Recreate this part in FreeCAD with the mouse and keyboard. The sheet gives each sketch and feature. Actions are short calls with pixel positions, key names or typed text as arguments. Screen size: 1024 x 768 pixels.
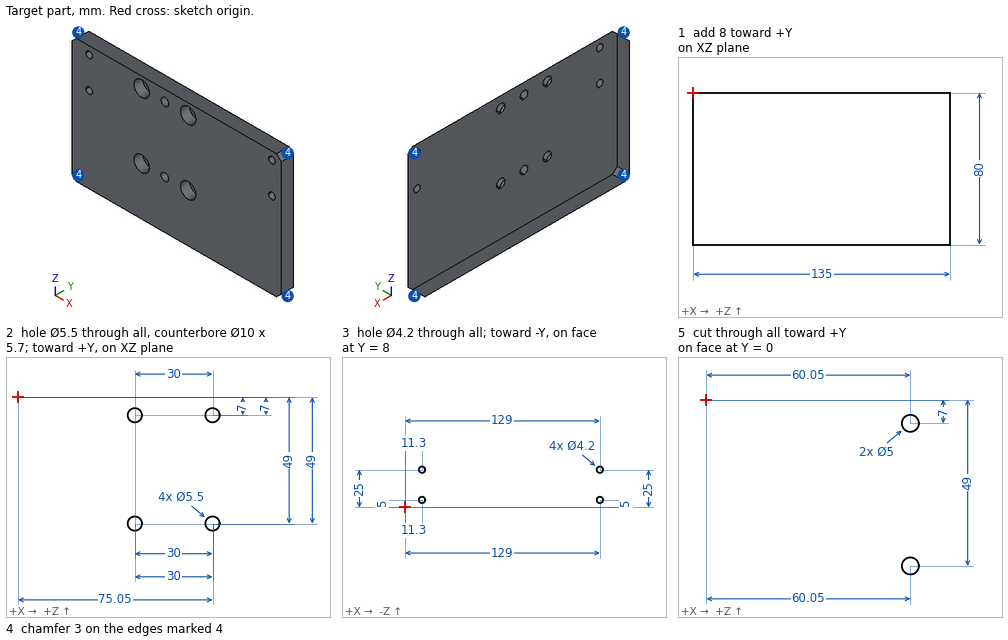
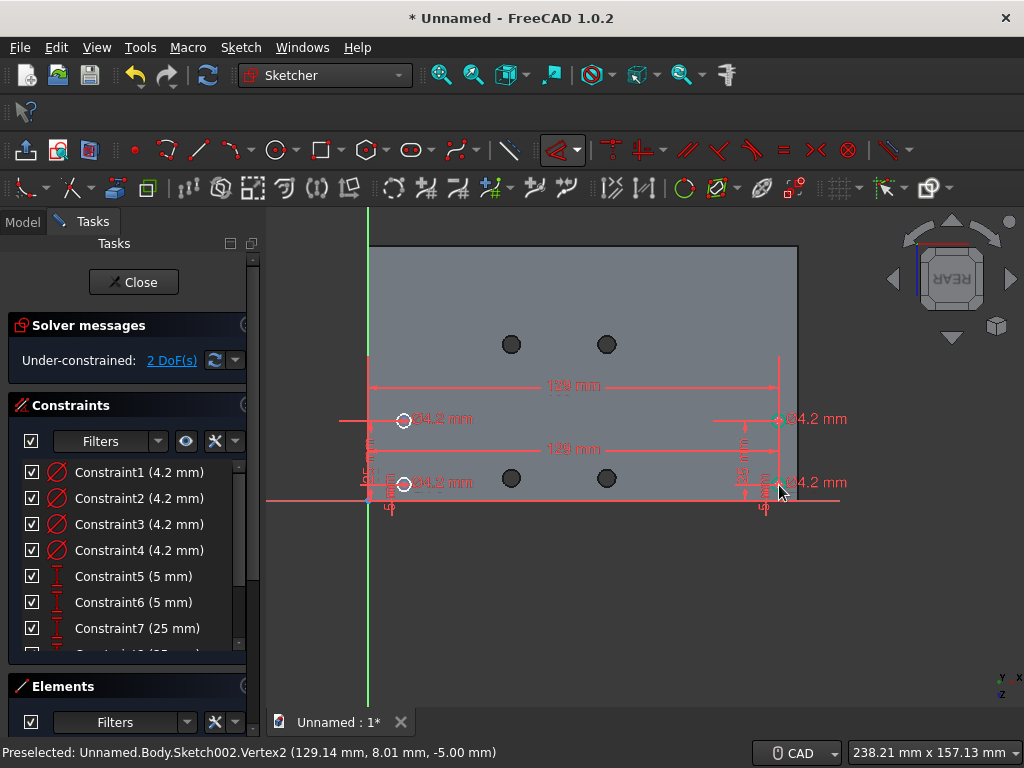
click(404, 421)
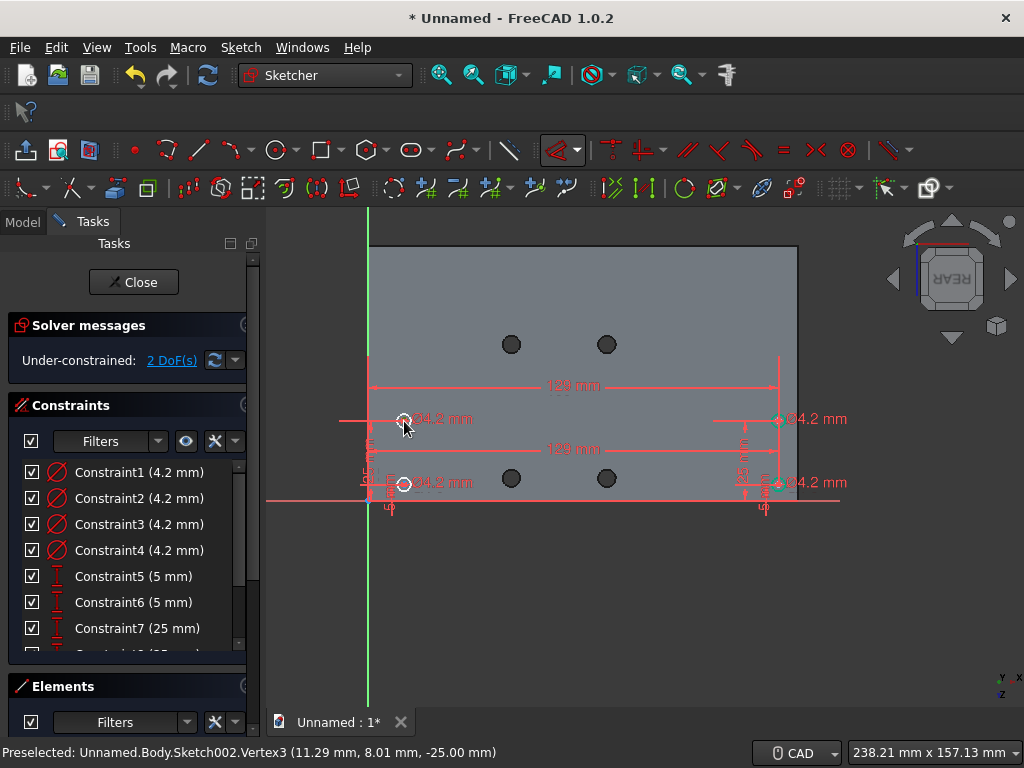
key(l)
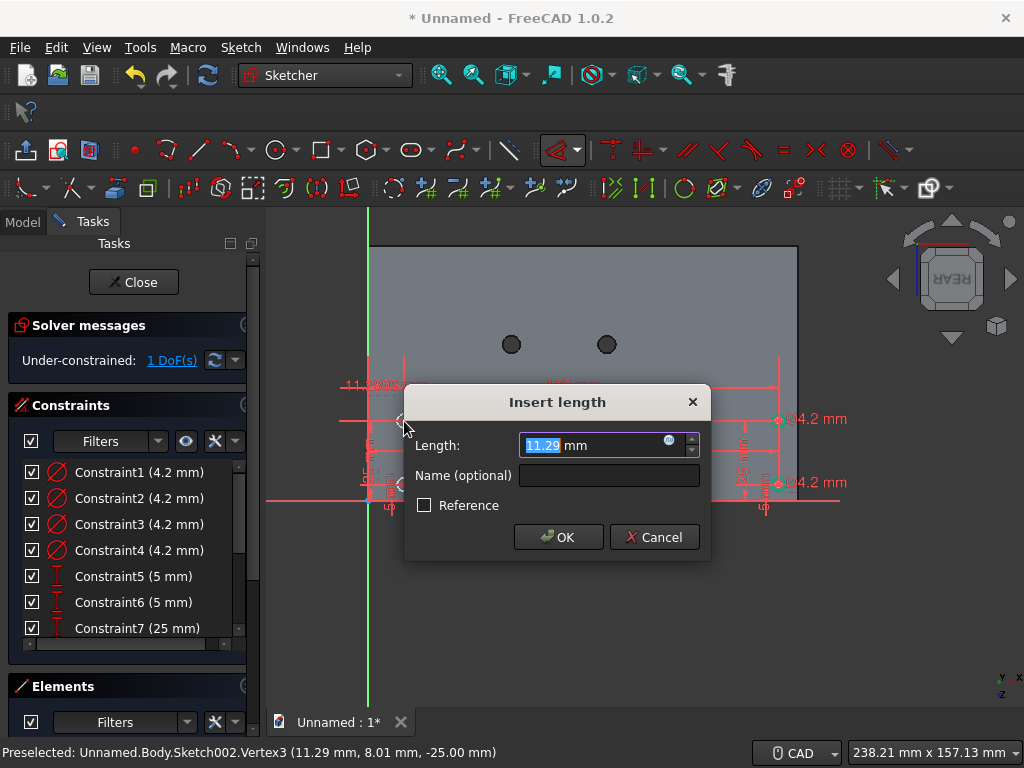
text(11.3)
key(Return)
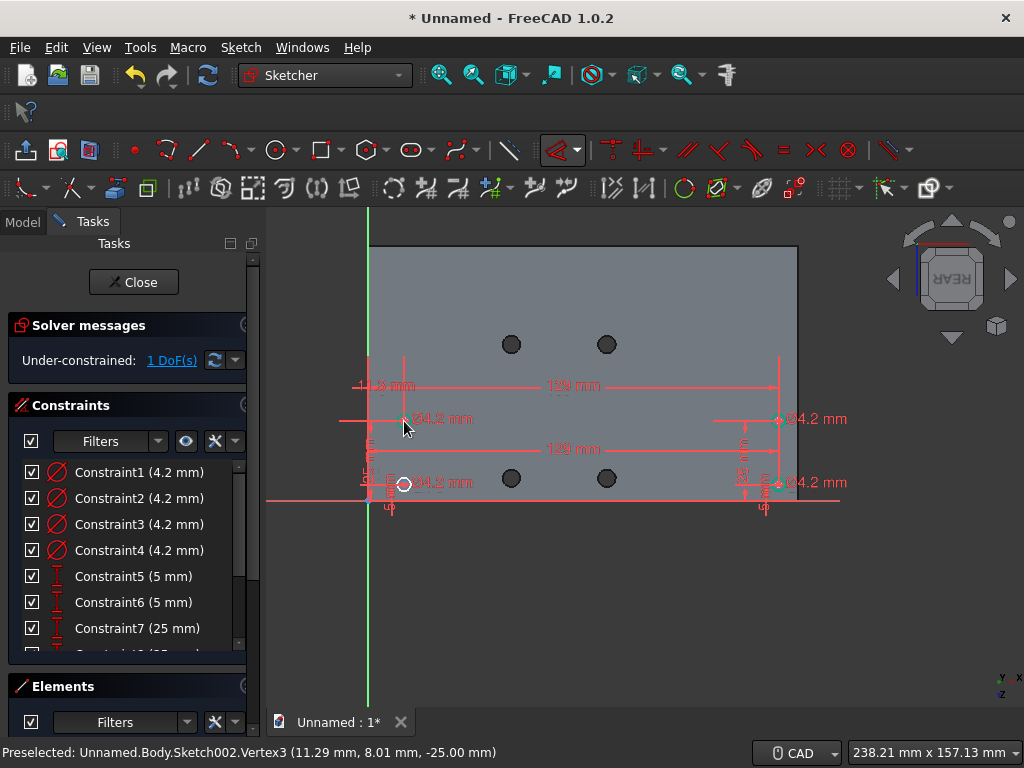
click(404, 485)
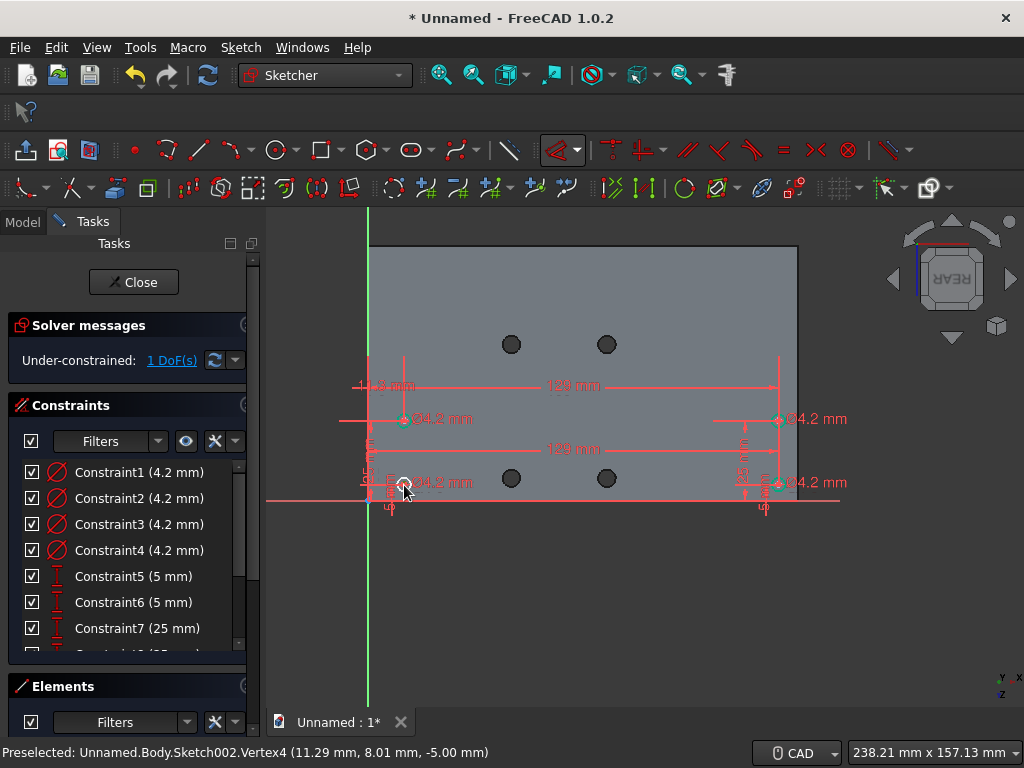
key(l)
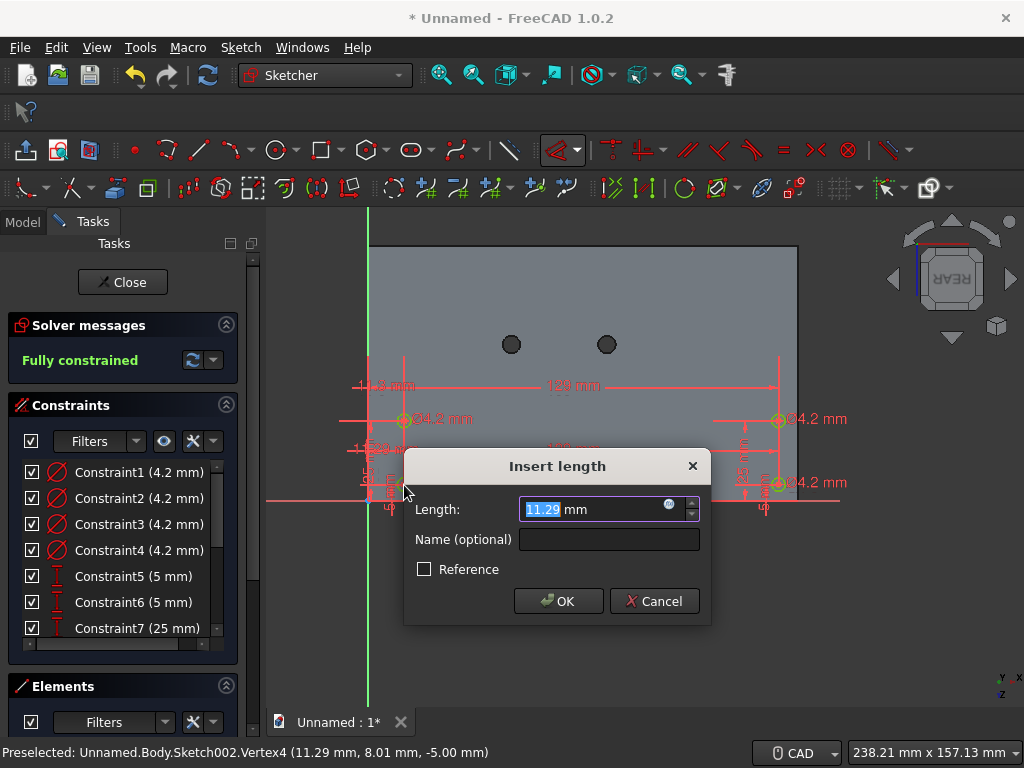
text(11.3)
key(Return)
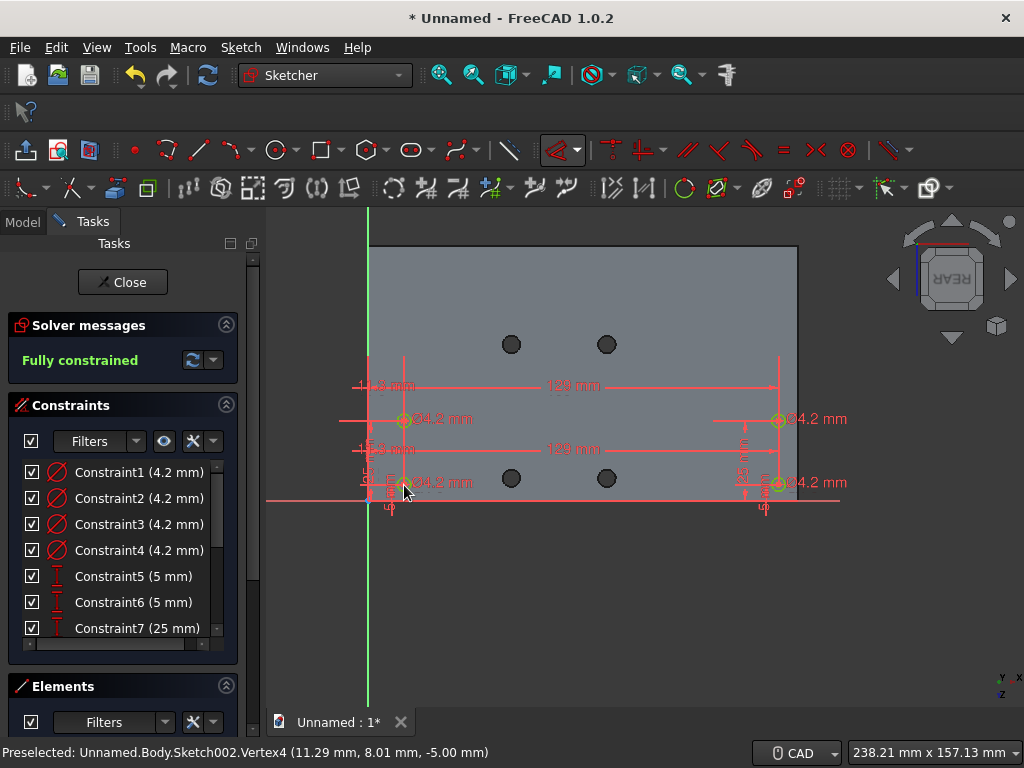
click(123, 282)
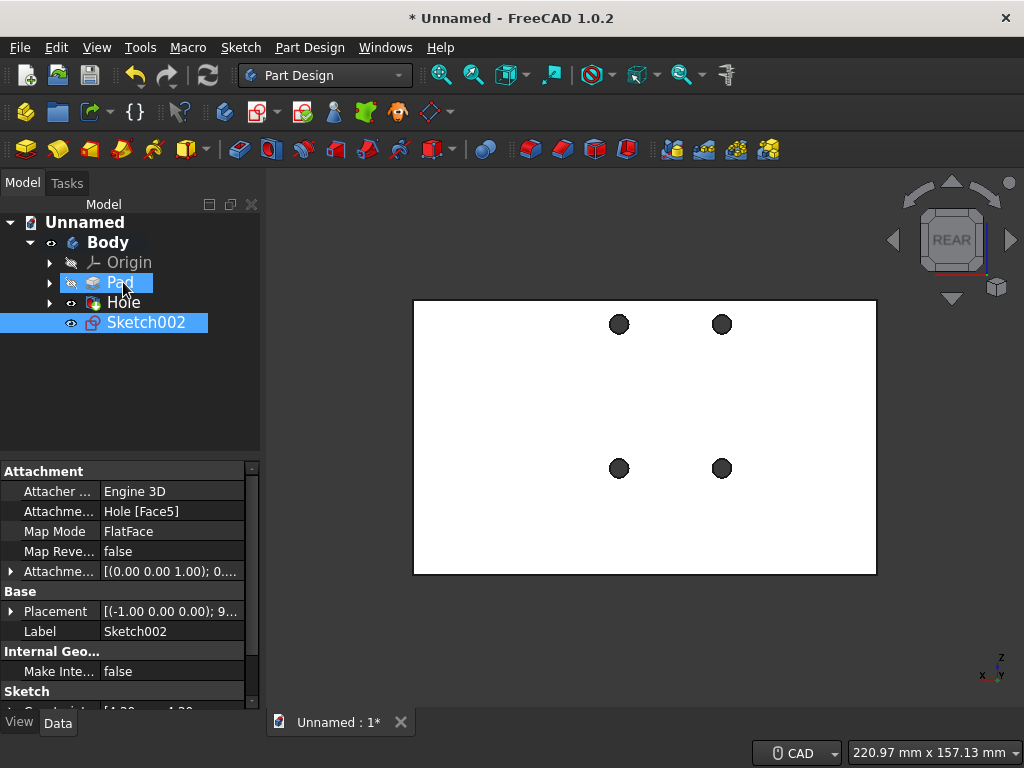
click(272, 150)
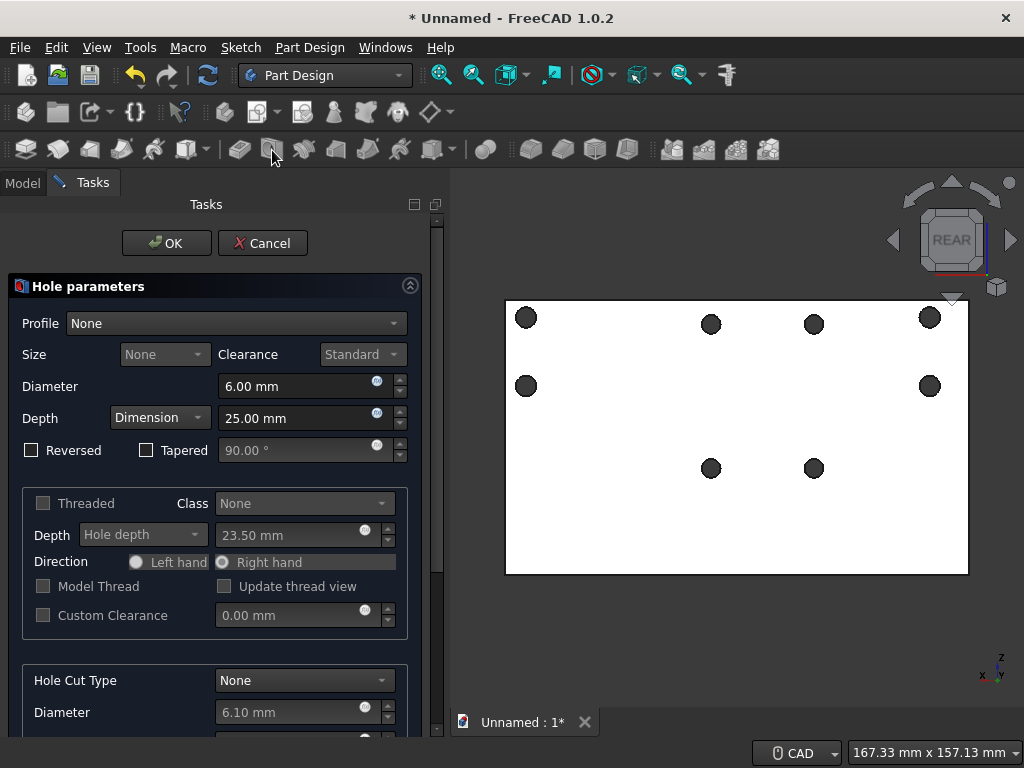
triple_click(305, 386)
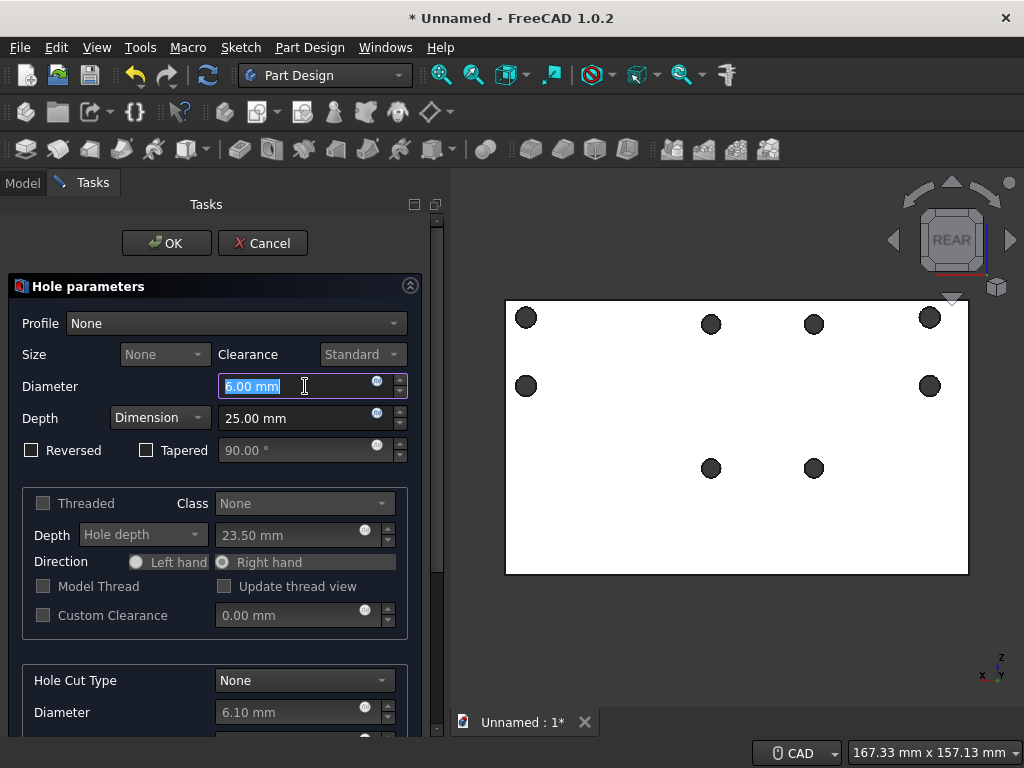
text(4.2)
key(Tab)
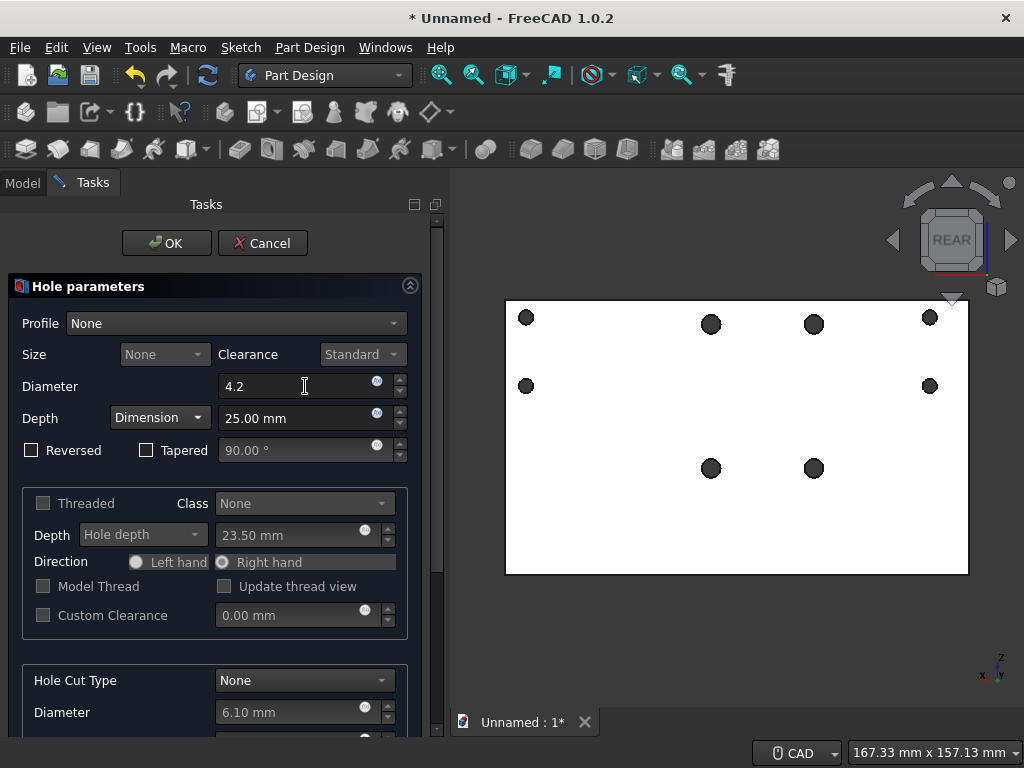
click(161, 418)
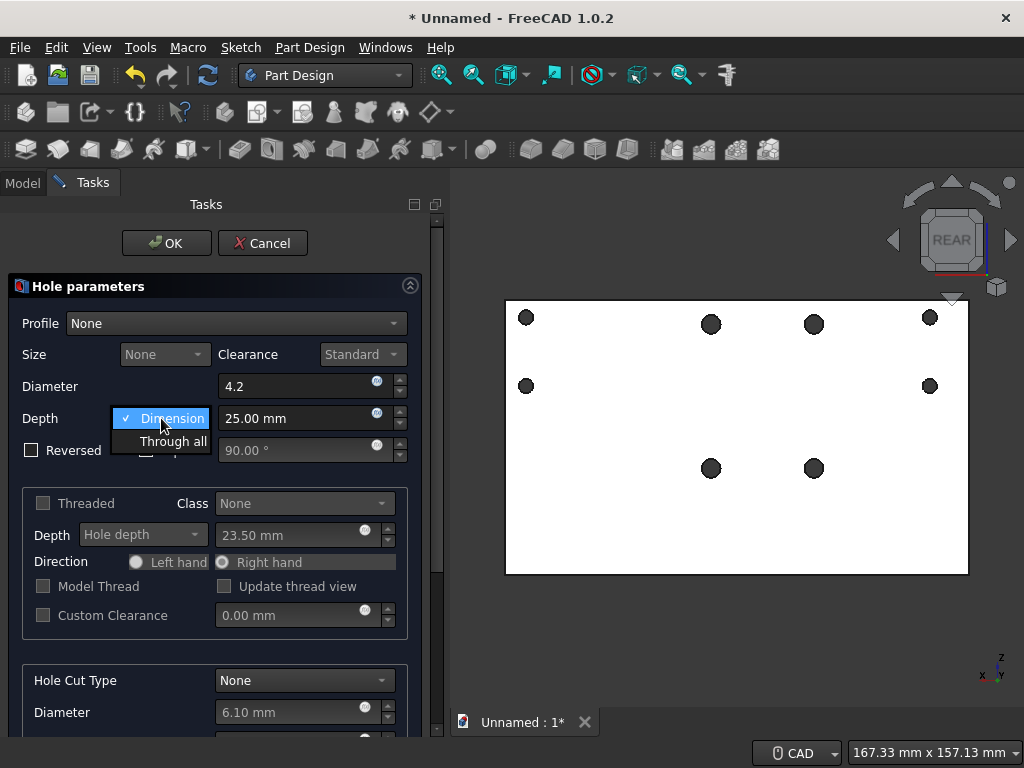
click(160, 442)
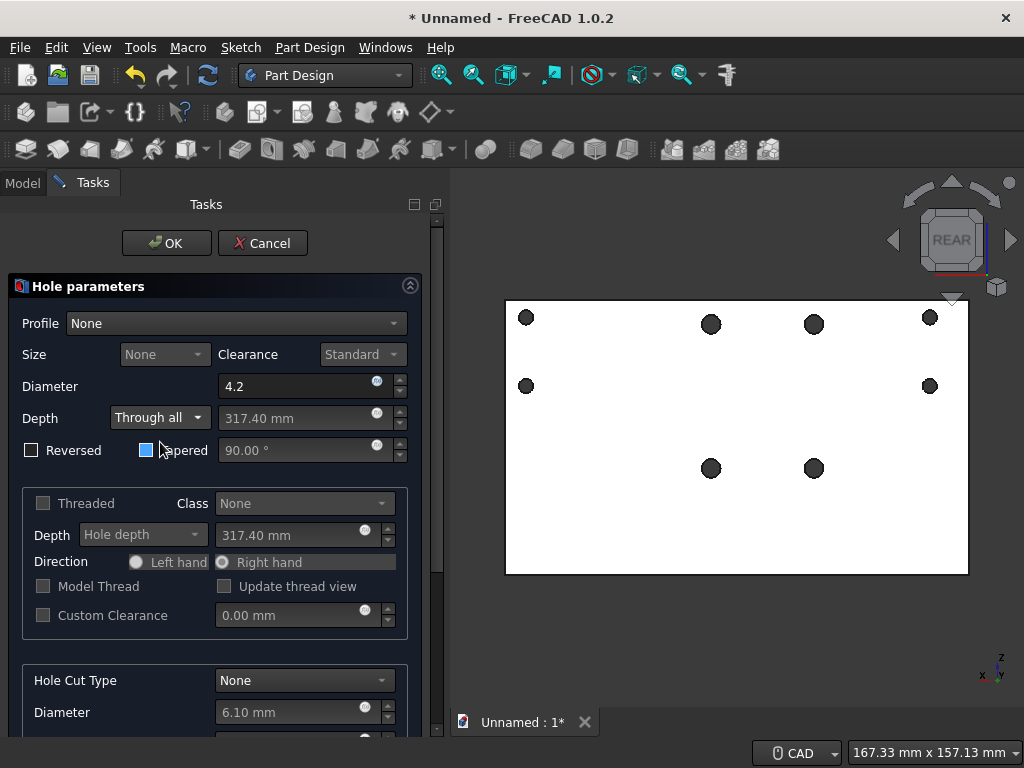
click(167, 243)